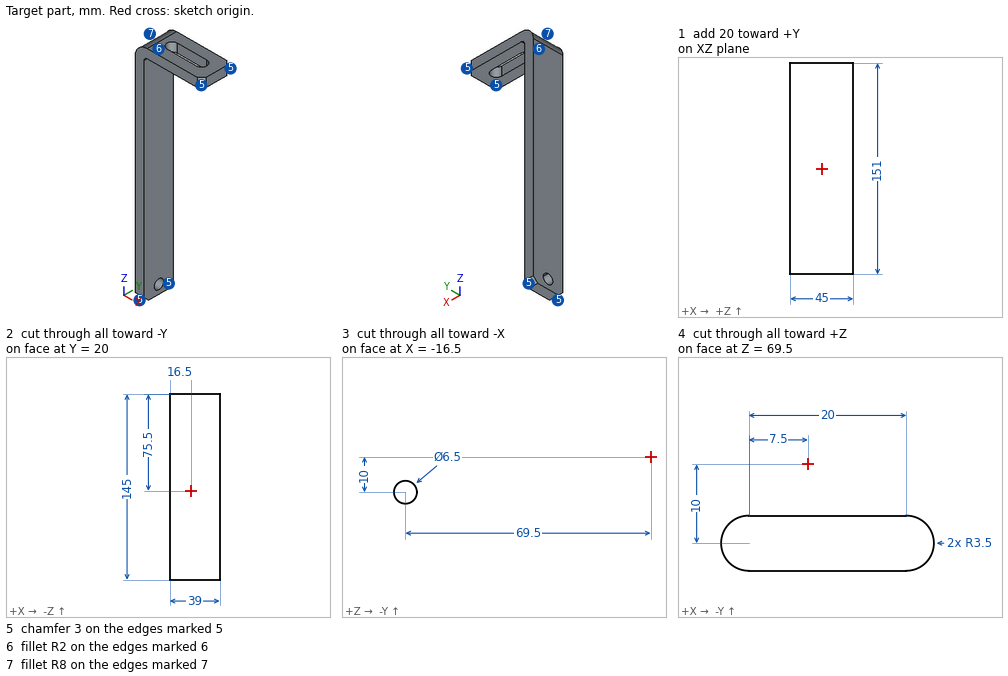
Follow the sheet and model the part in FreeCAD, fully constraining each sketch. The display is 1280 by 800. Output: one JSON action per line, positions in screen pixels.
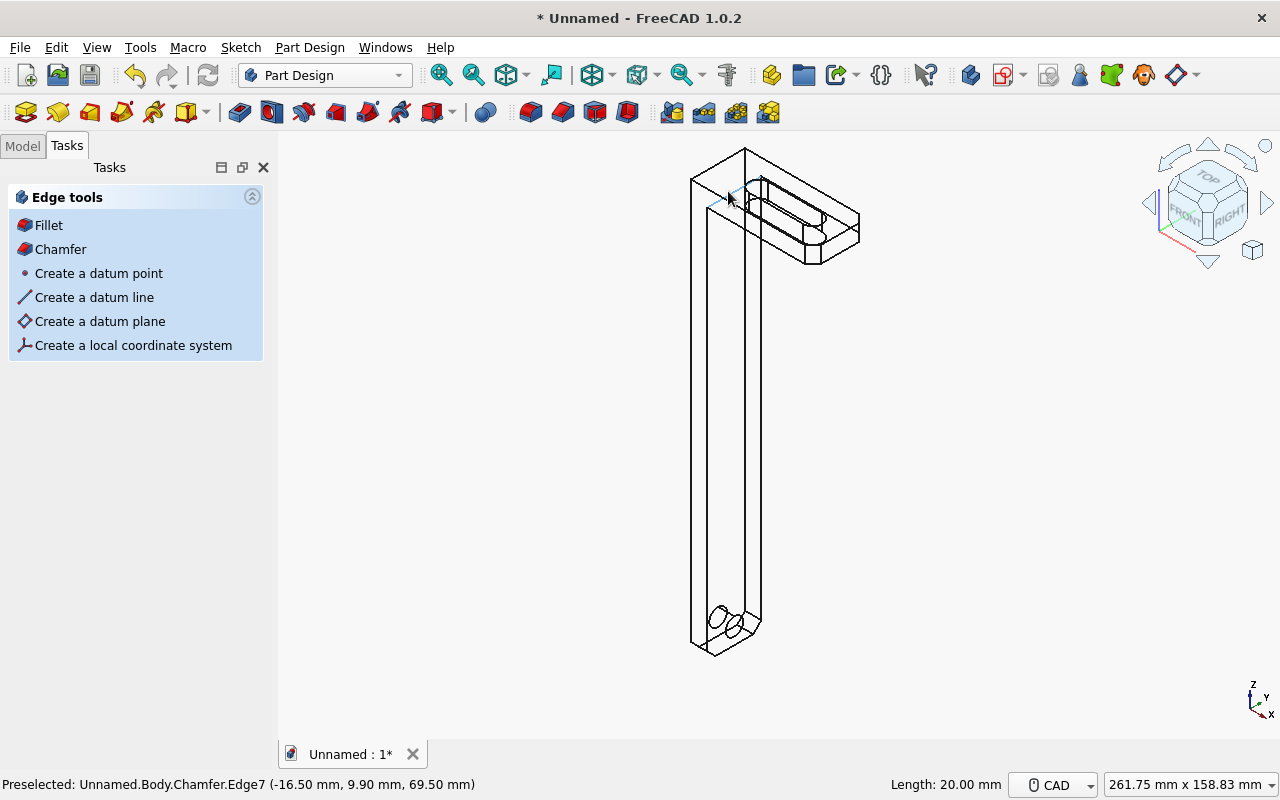
{"action": "key", "text": "v 1"}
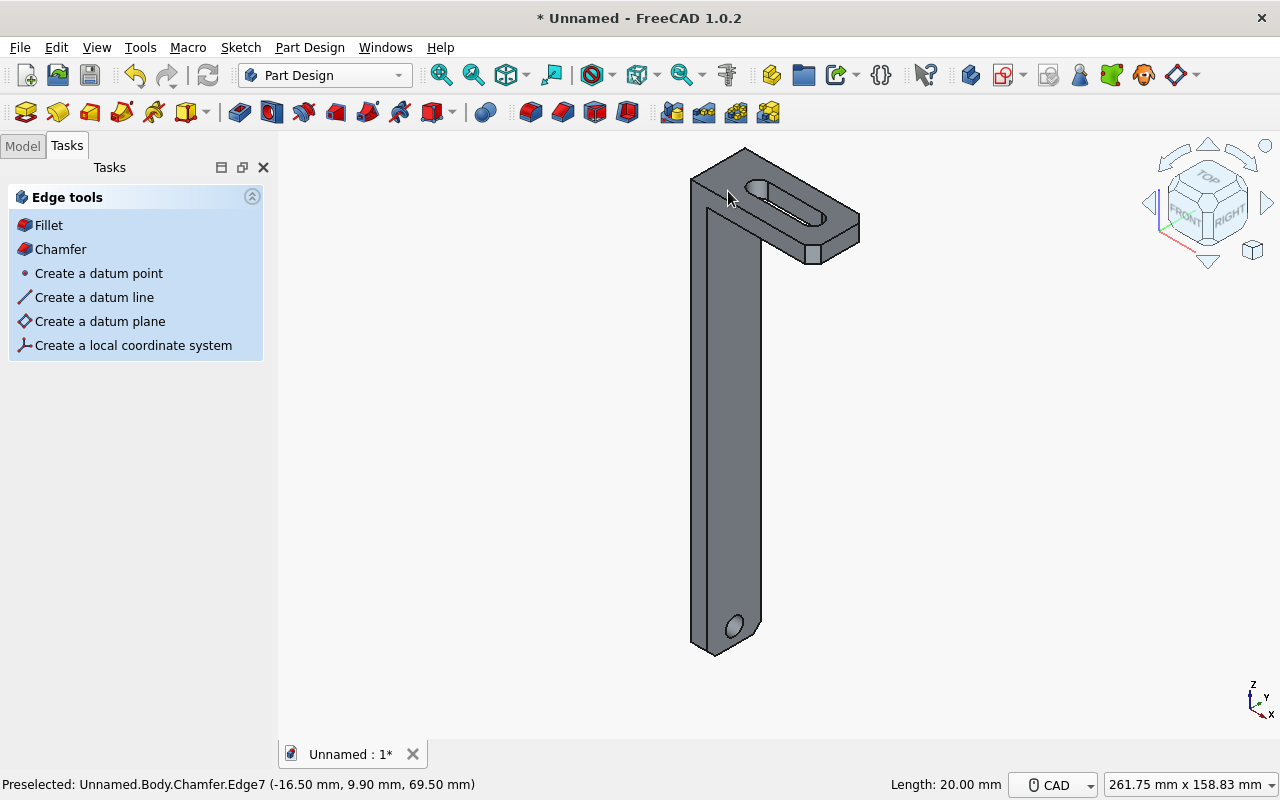
{"action": "left_click", "coordinate": [532, 112]}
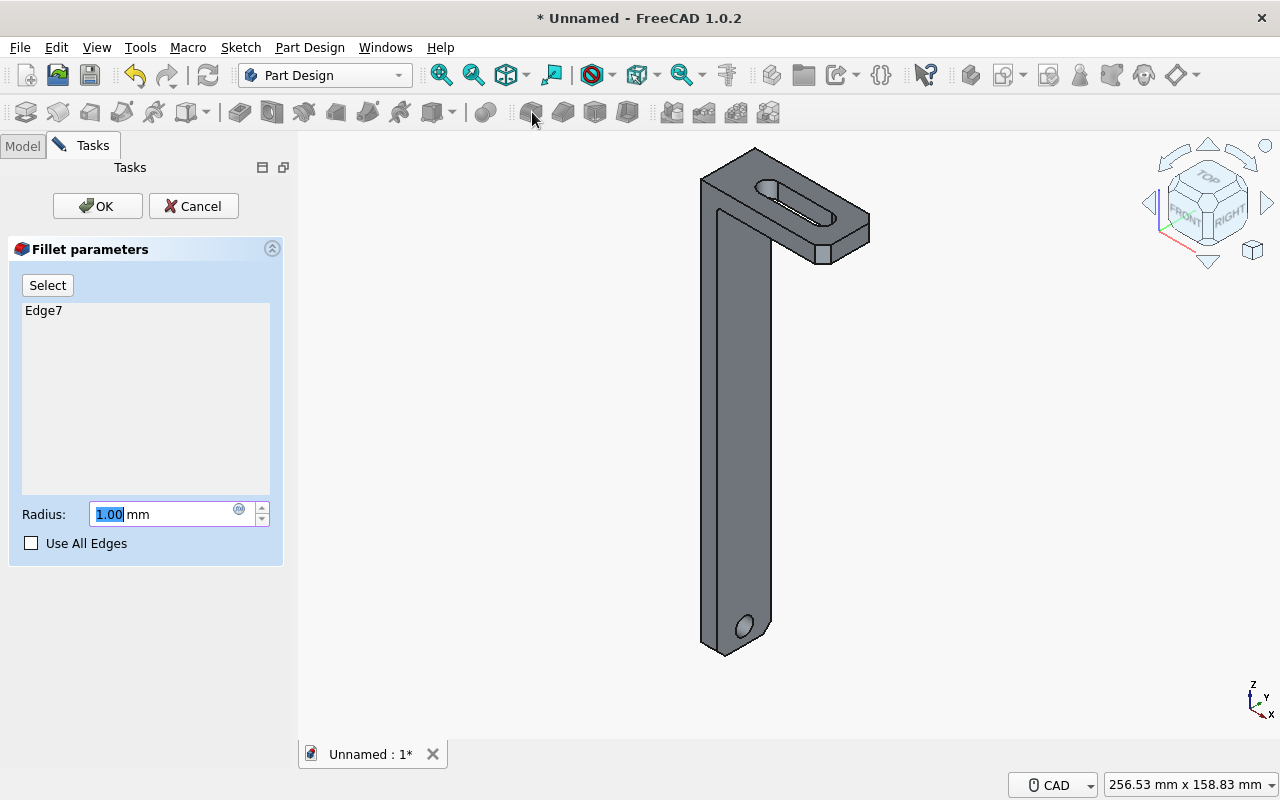
{"action": "type", "text": "2"}
{"action": "key", "text": "Tab"}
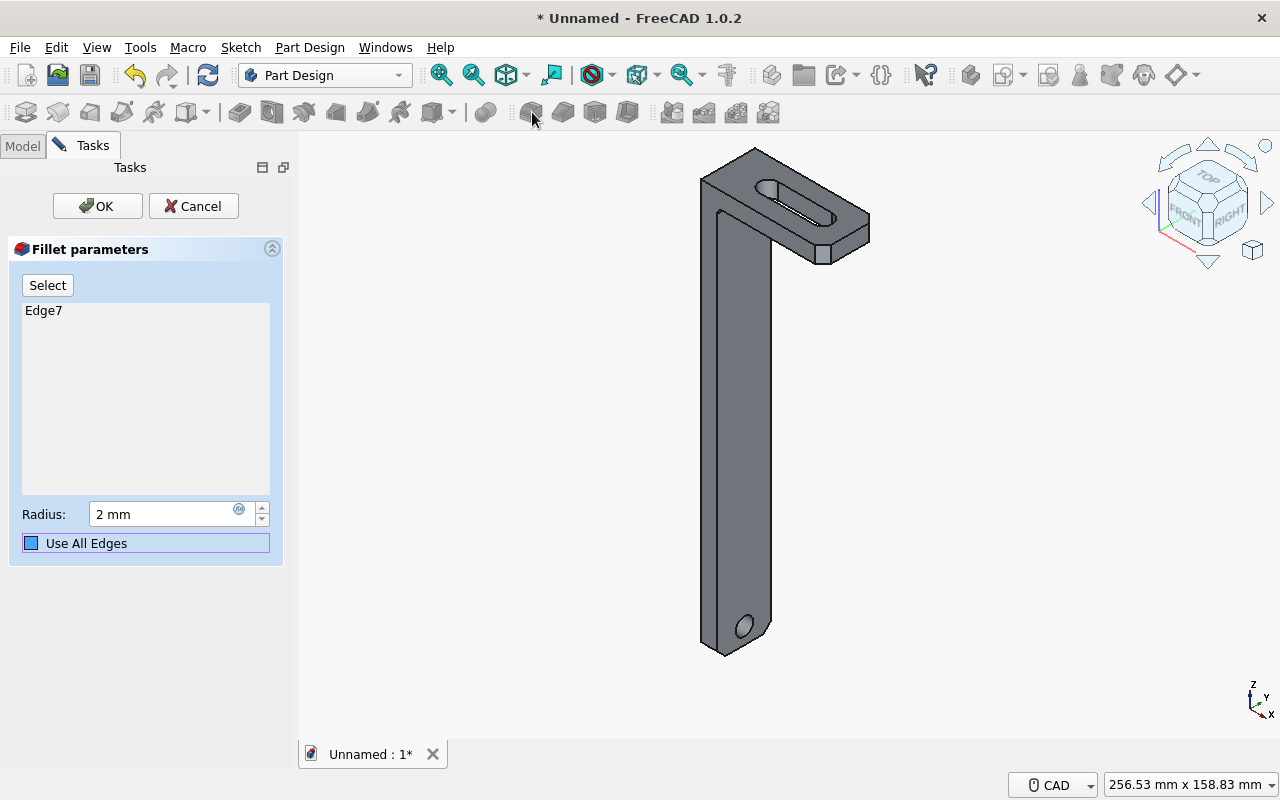
{"action": "left_click", "coordinate": [98, 206]}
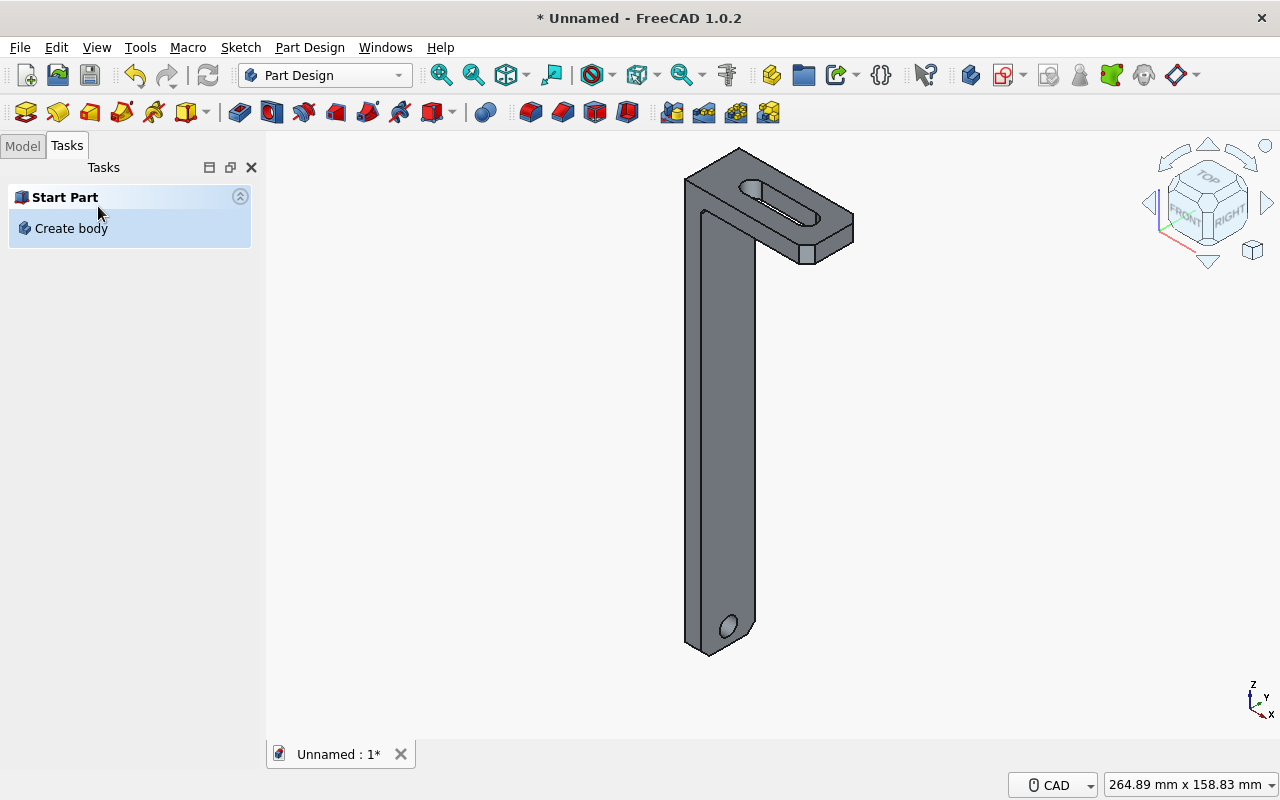
{"action": "key", "text": "2"}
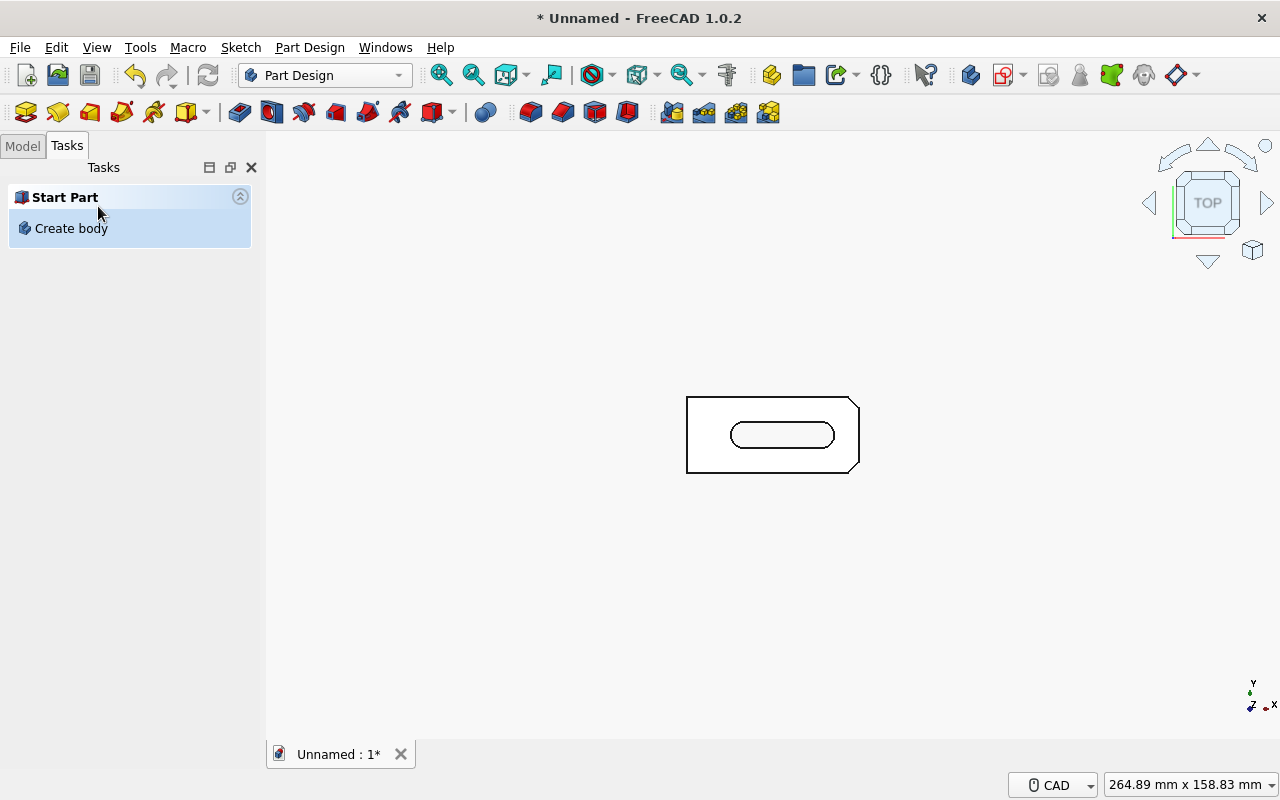
{"action": "left_click", "coordinate": [442, 76]}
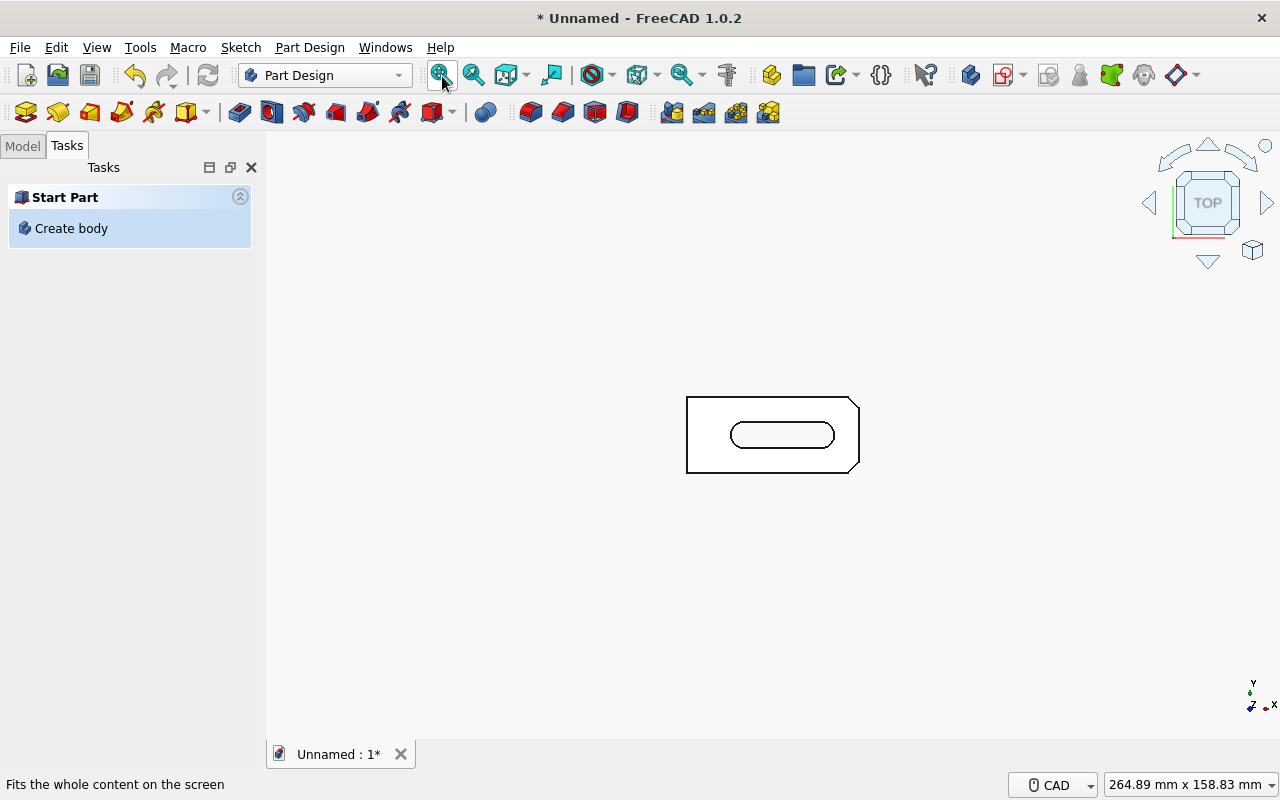
{"action": "left_click", "coordinate": [687, 434]}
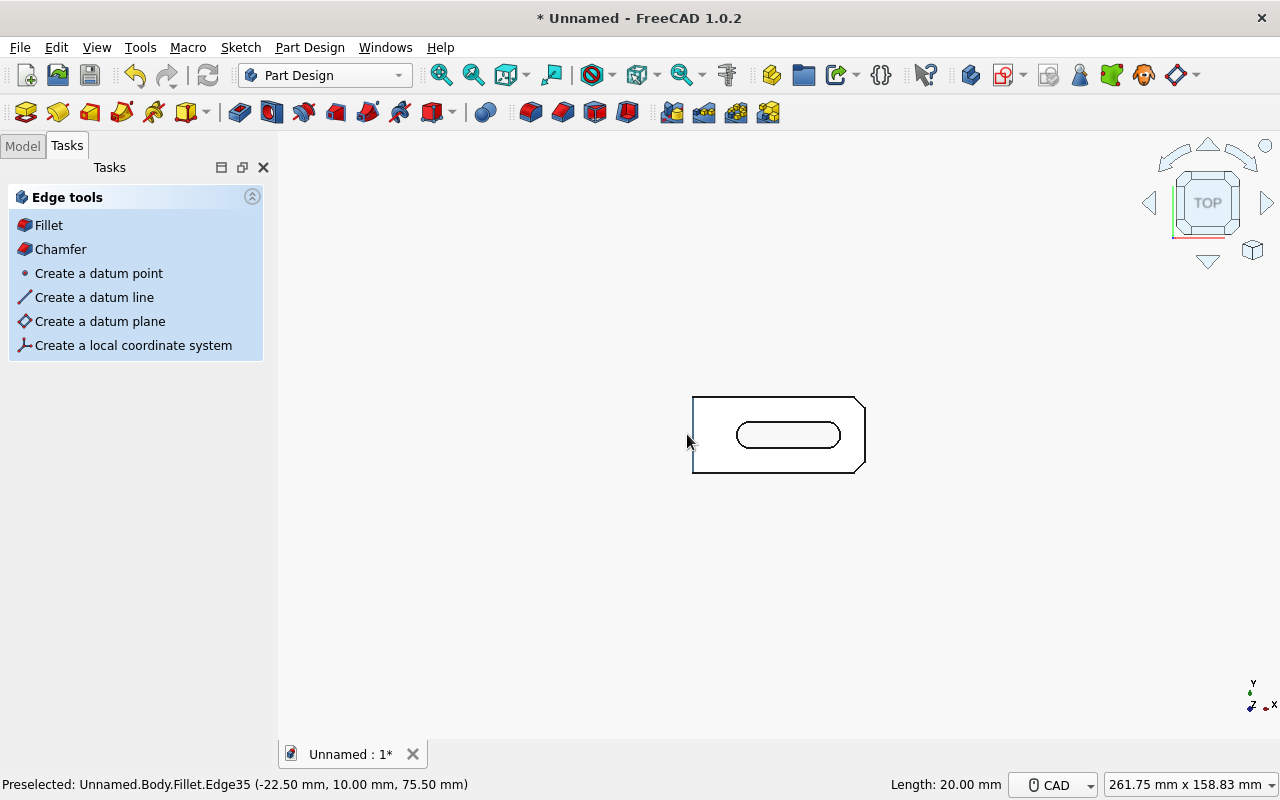
{"action": "left_click", "coordinate": [532, 112]}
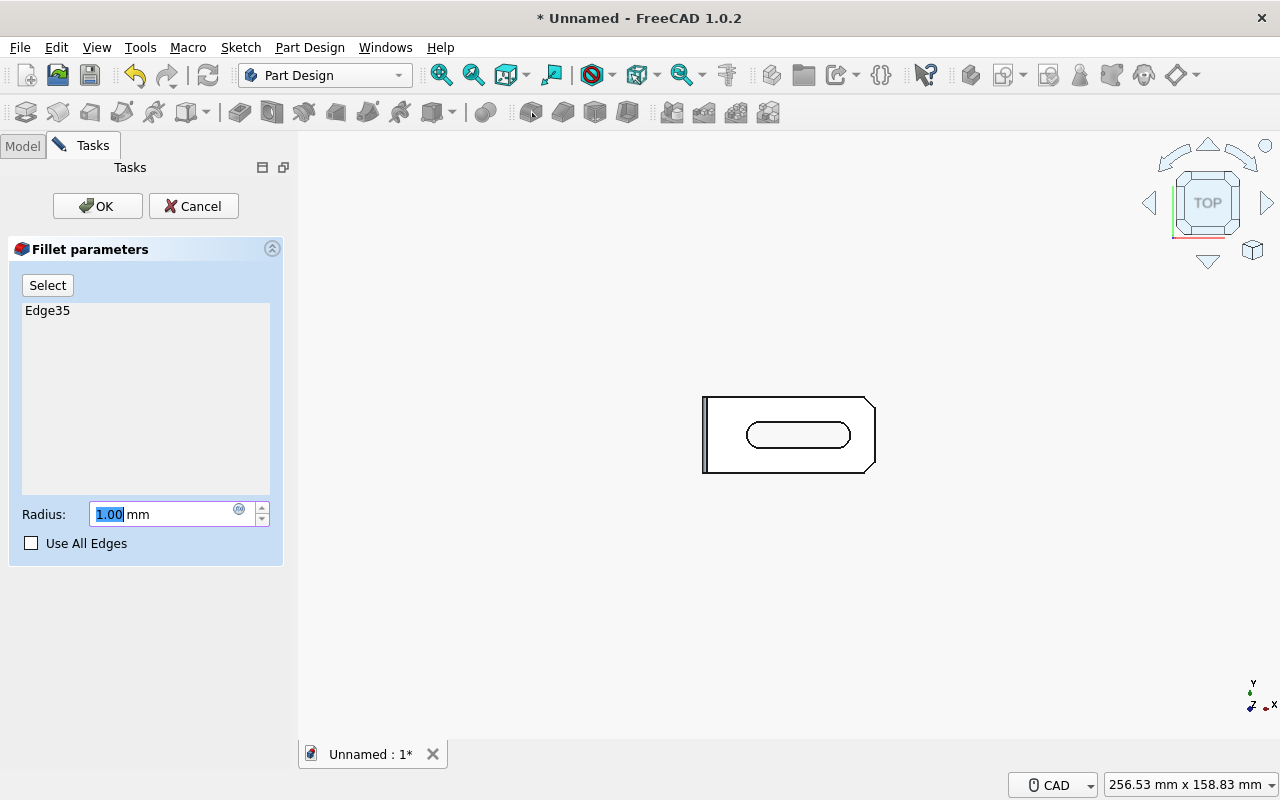
{"action": "type", "text": "8"}
{"action": "key", "text": "Tab"}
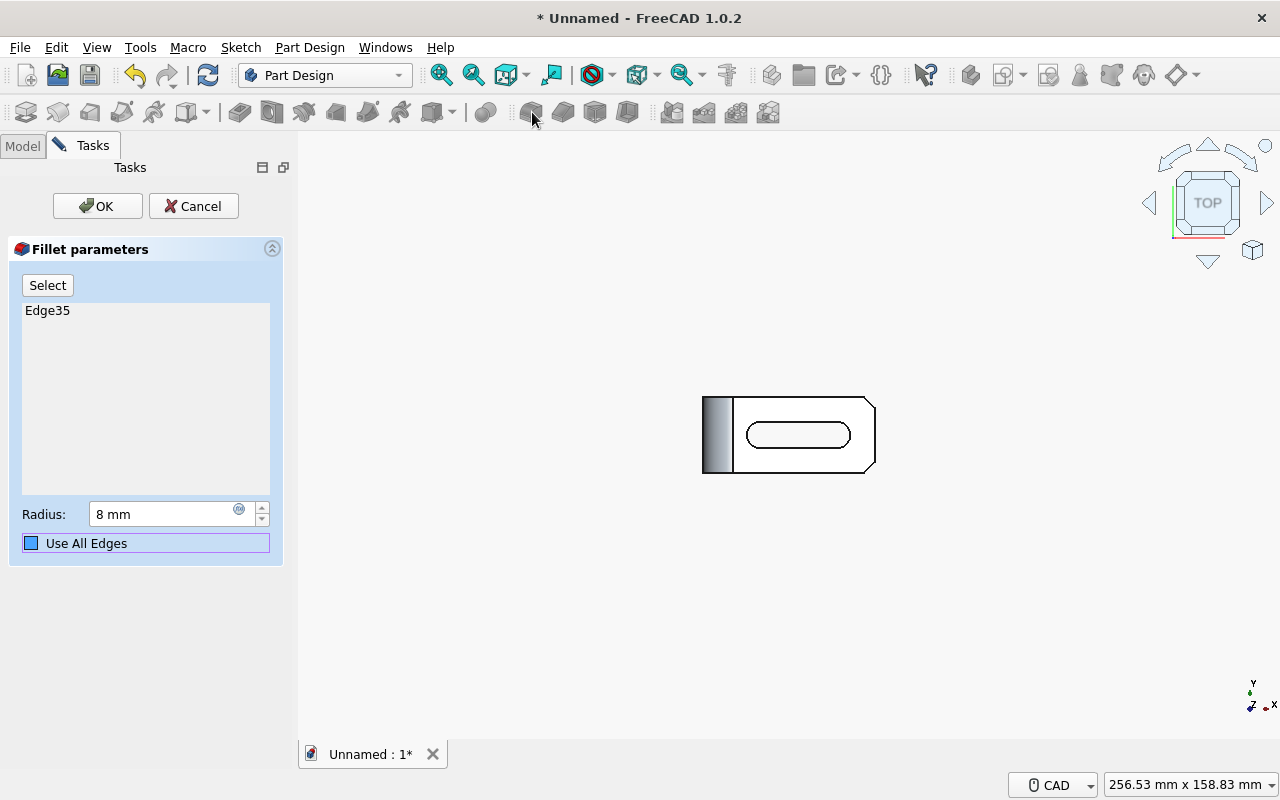
{"action": "left_click", "coordinate": [98, 206]}